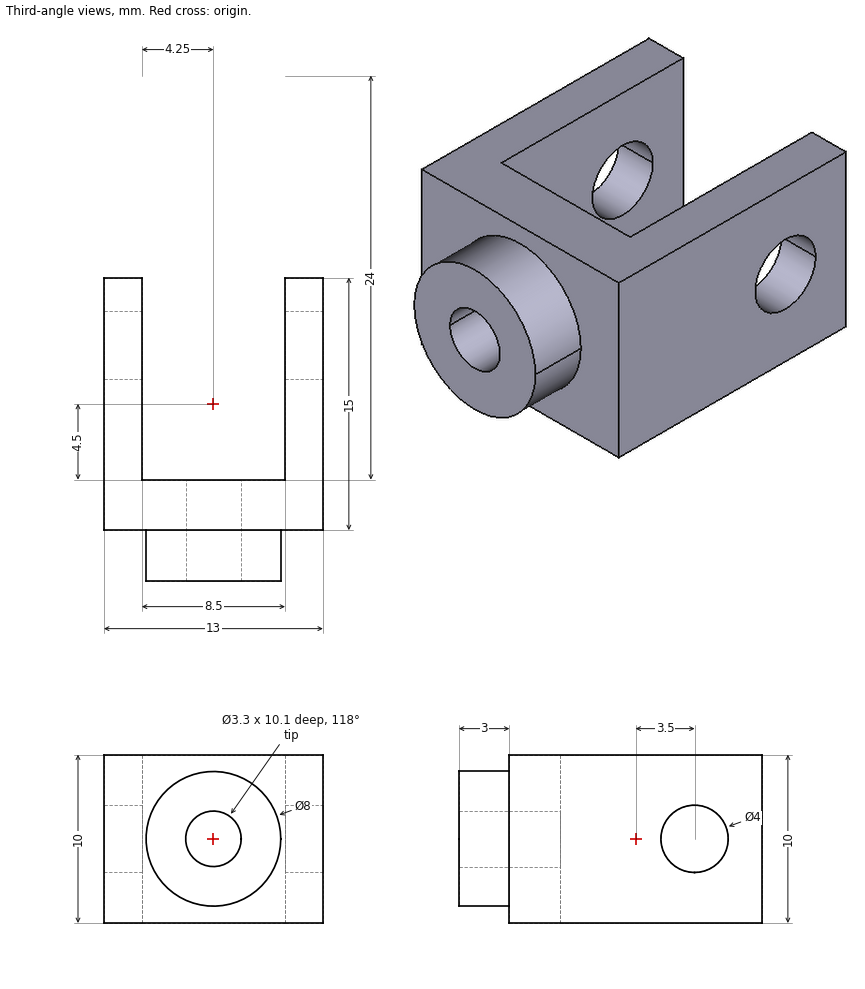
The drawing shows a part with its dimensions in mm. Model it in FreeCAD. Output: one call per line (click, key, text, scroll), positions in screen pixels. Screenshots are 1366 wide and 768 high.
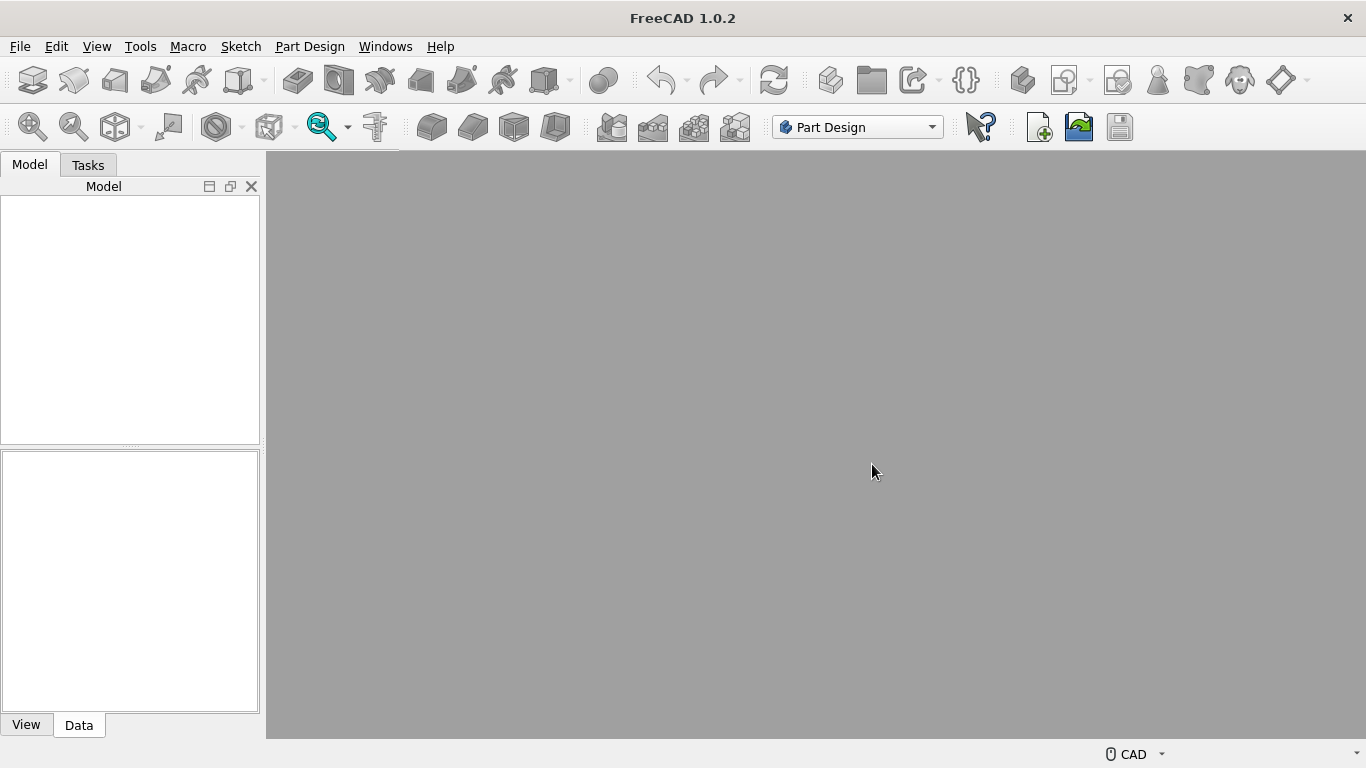
click(1038, 128)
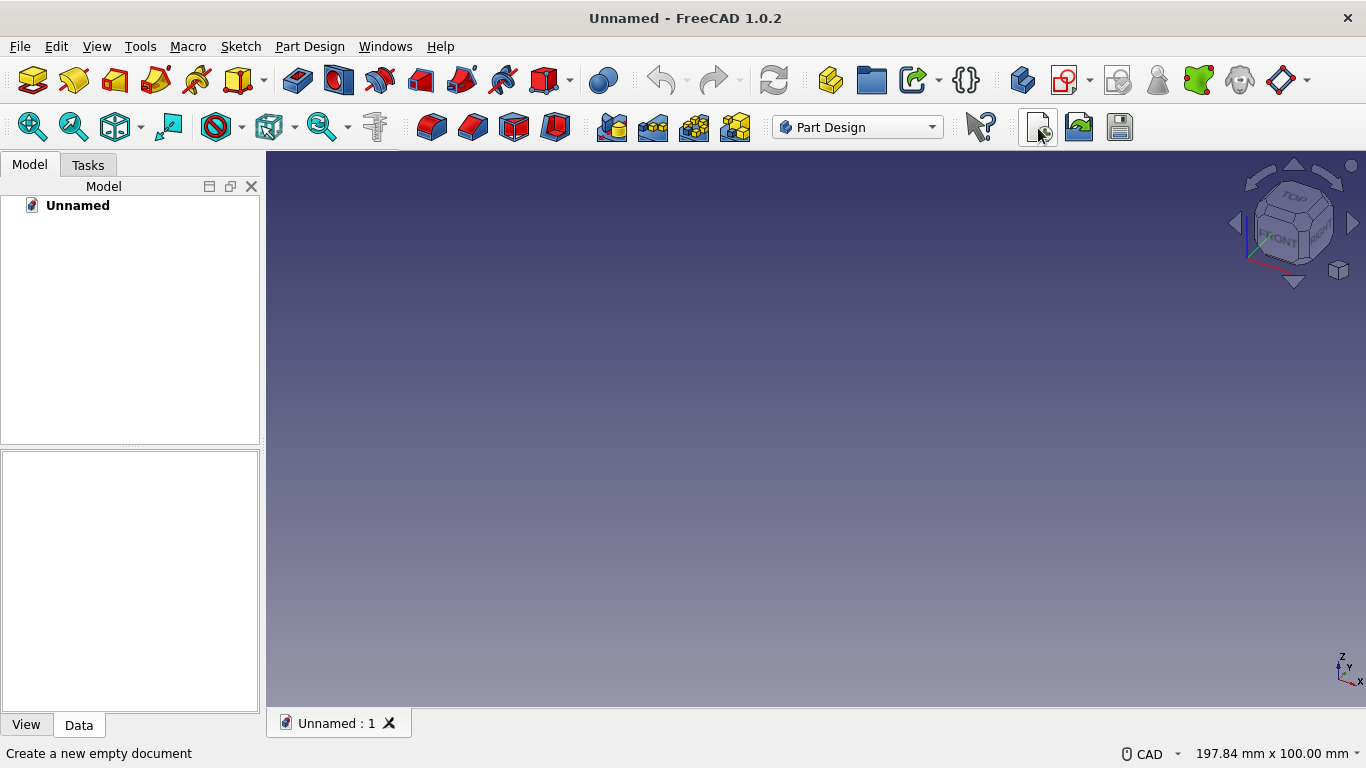
click(1064, 80)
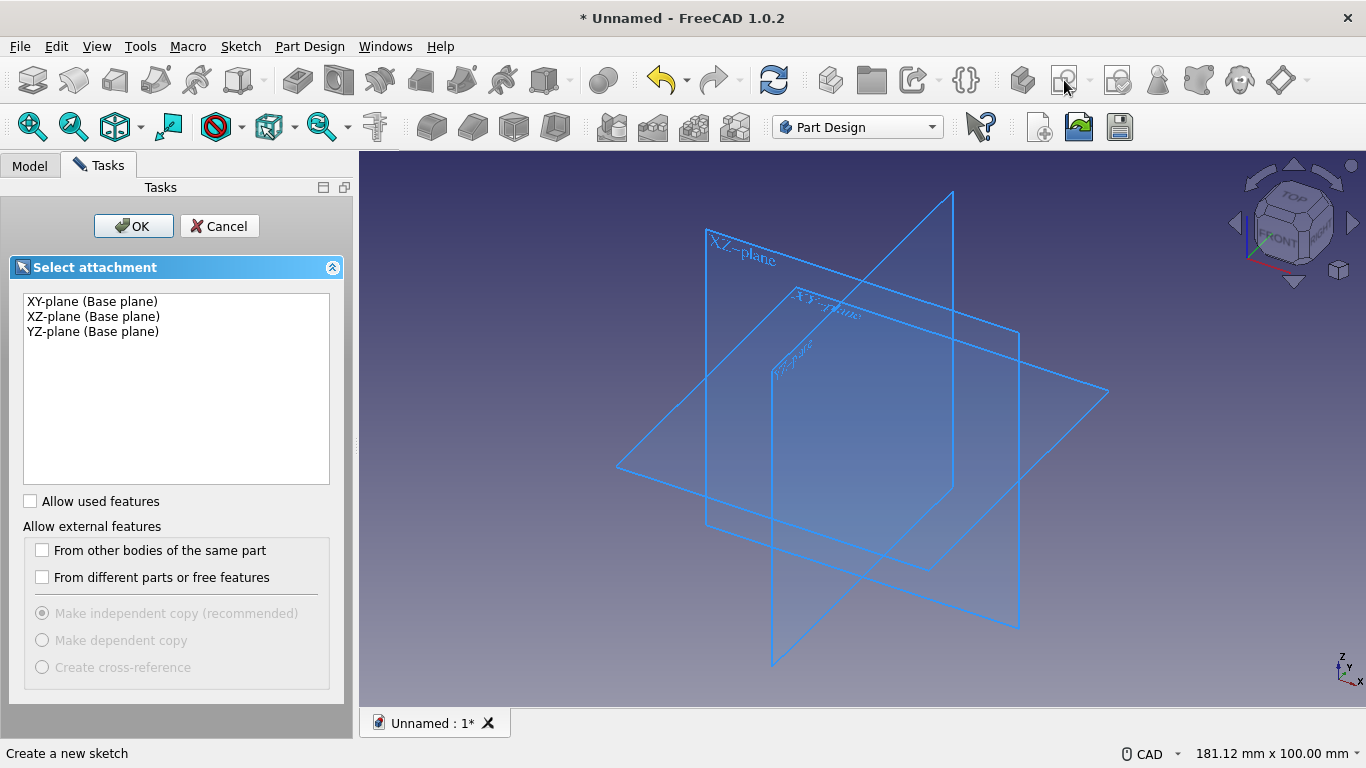
click(84, 302)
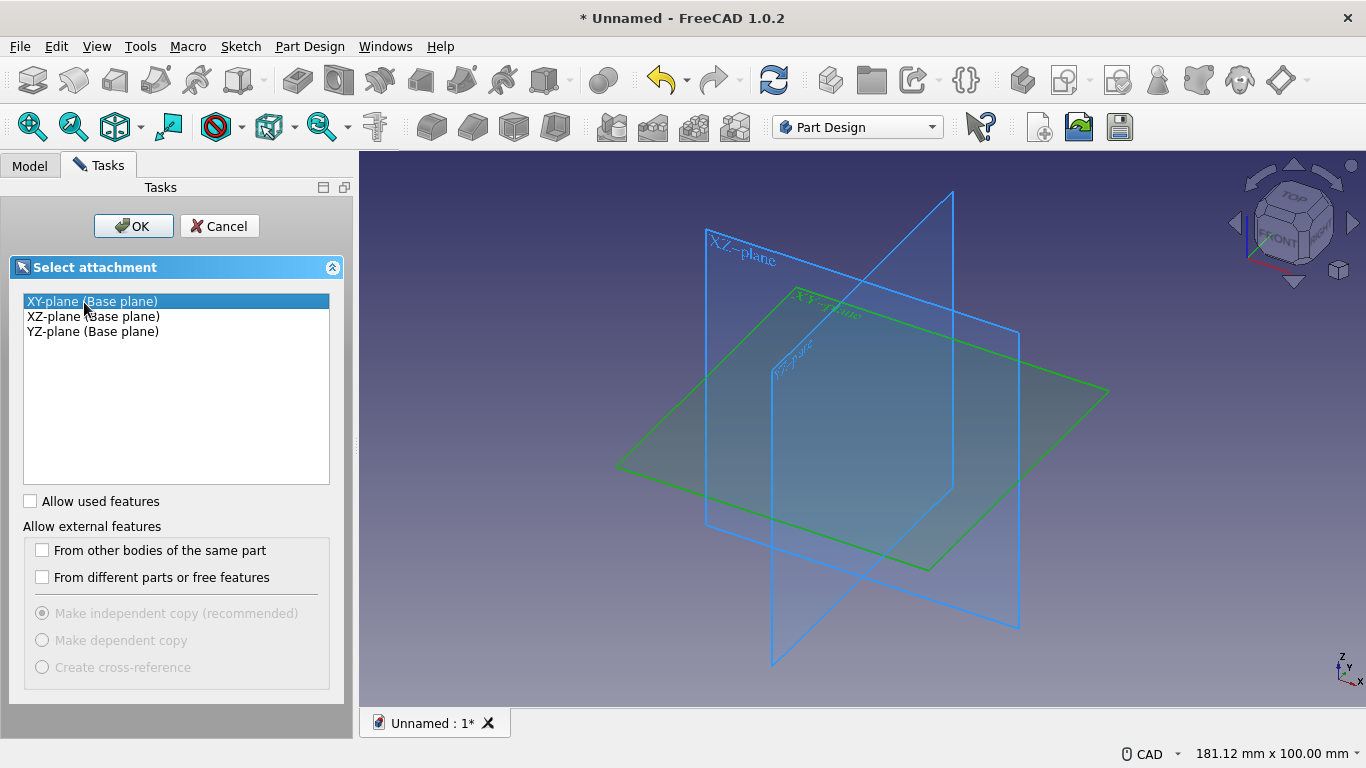
click(134, 226)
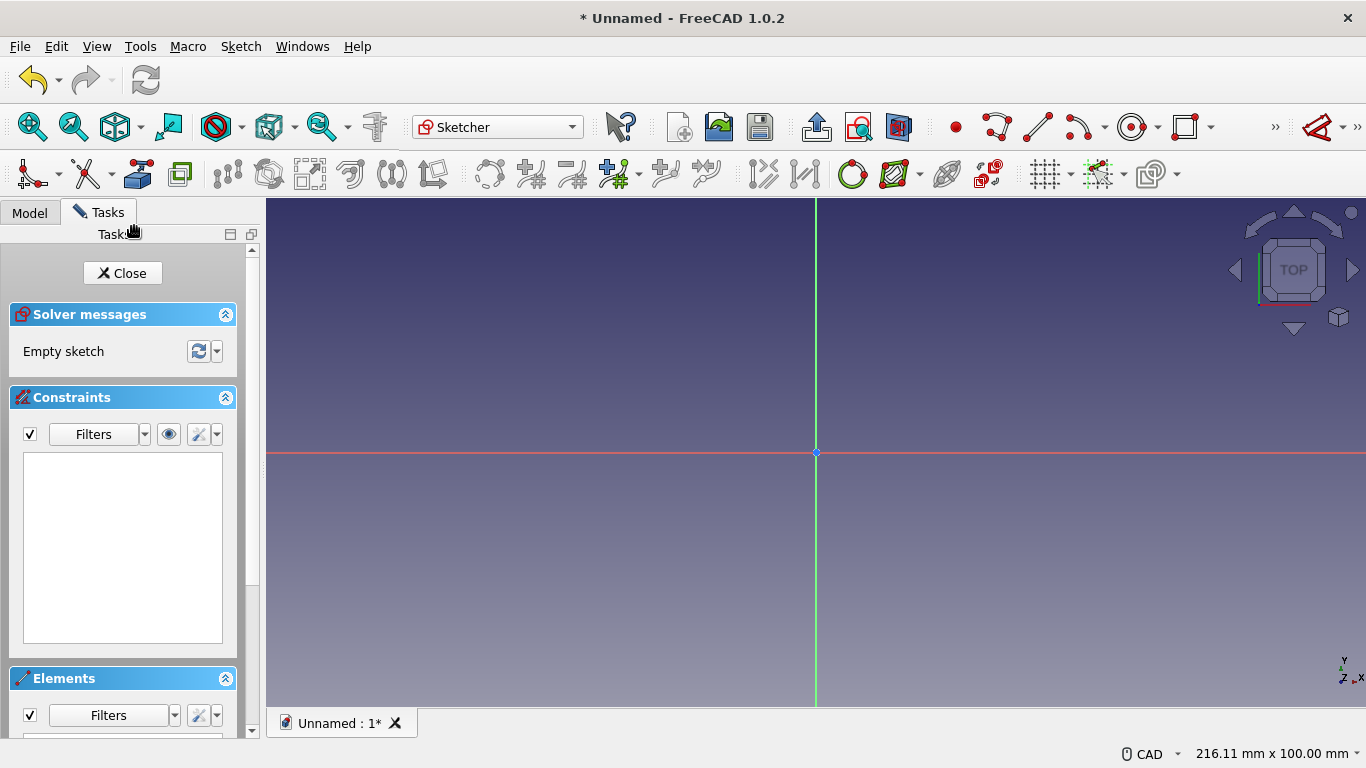
scroll(838, 452, up, 7)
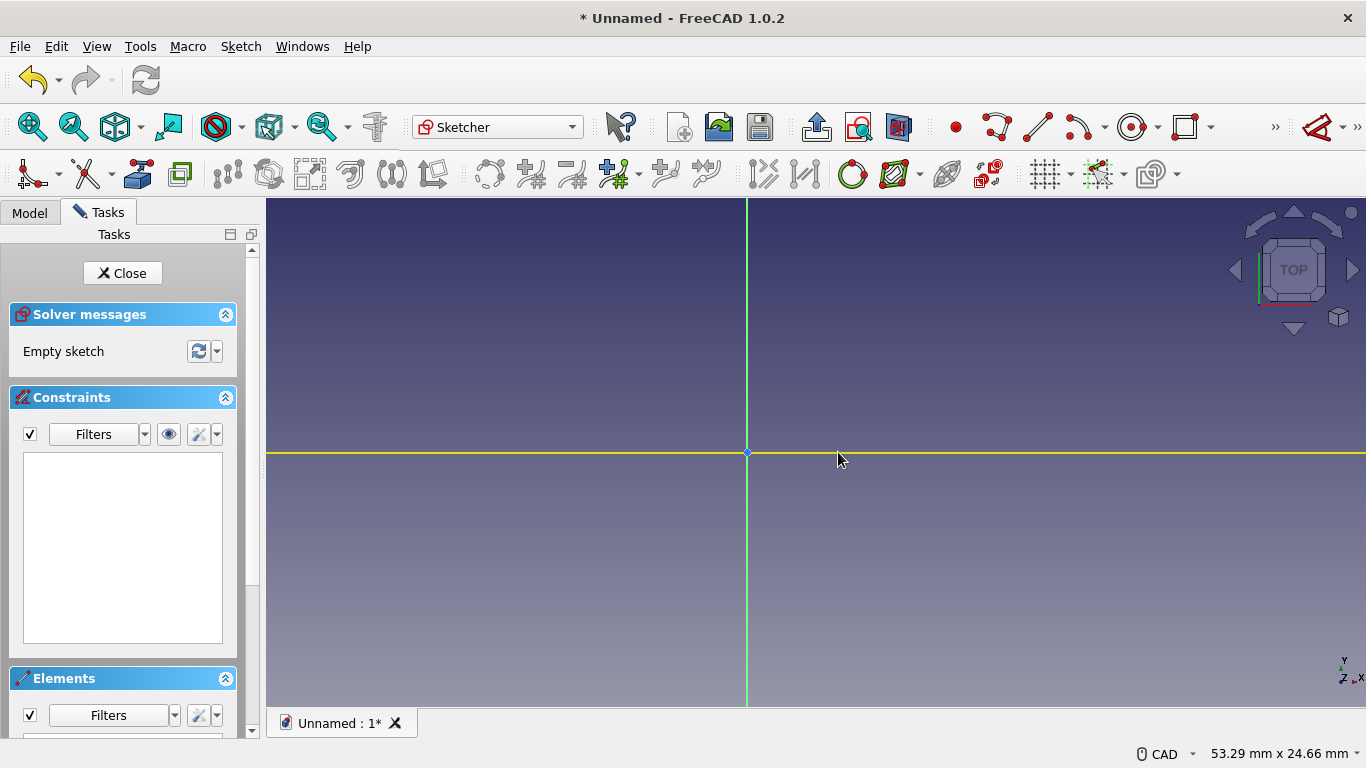
key(g)
key(v)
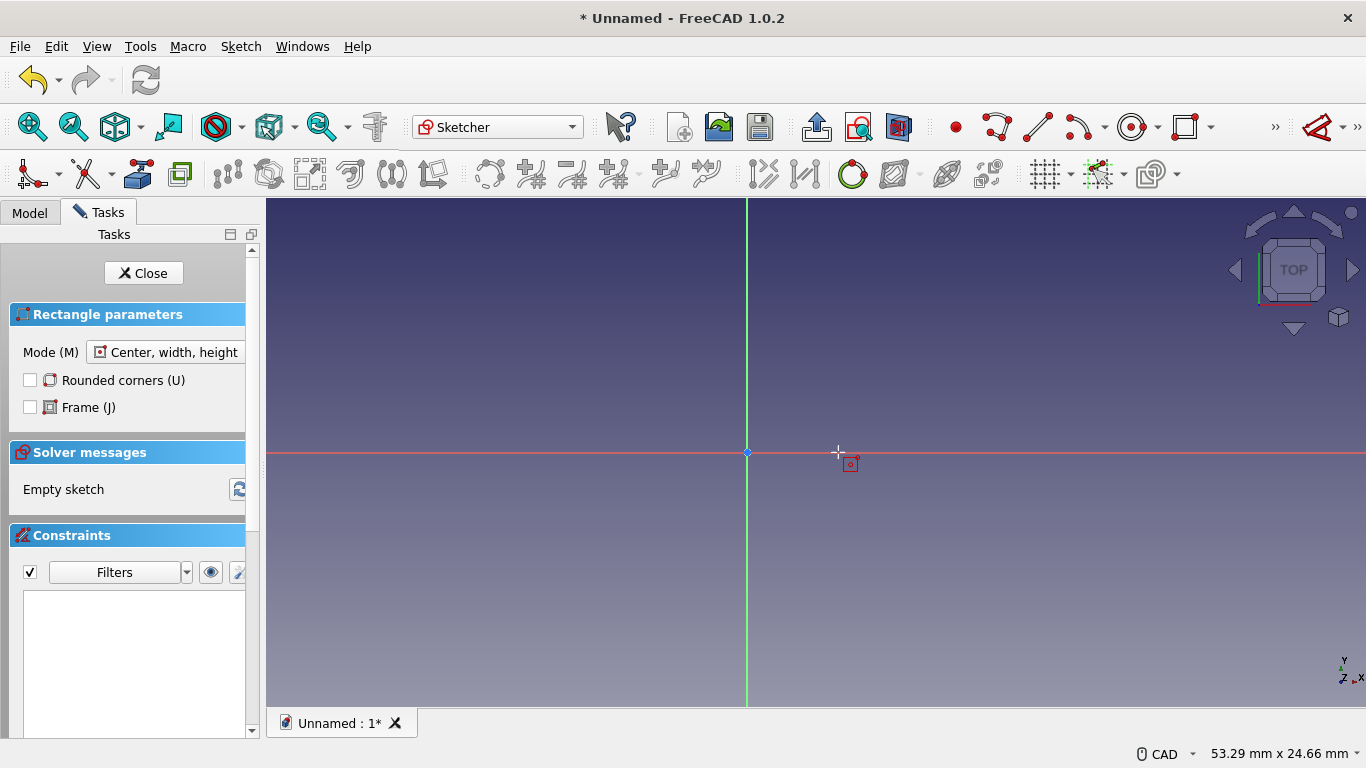
click(747, 452)
move(881, 298)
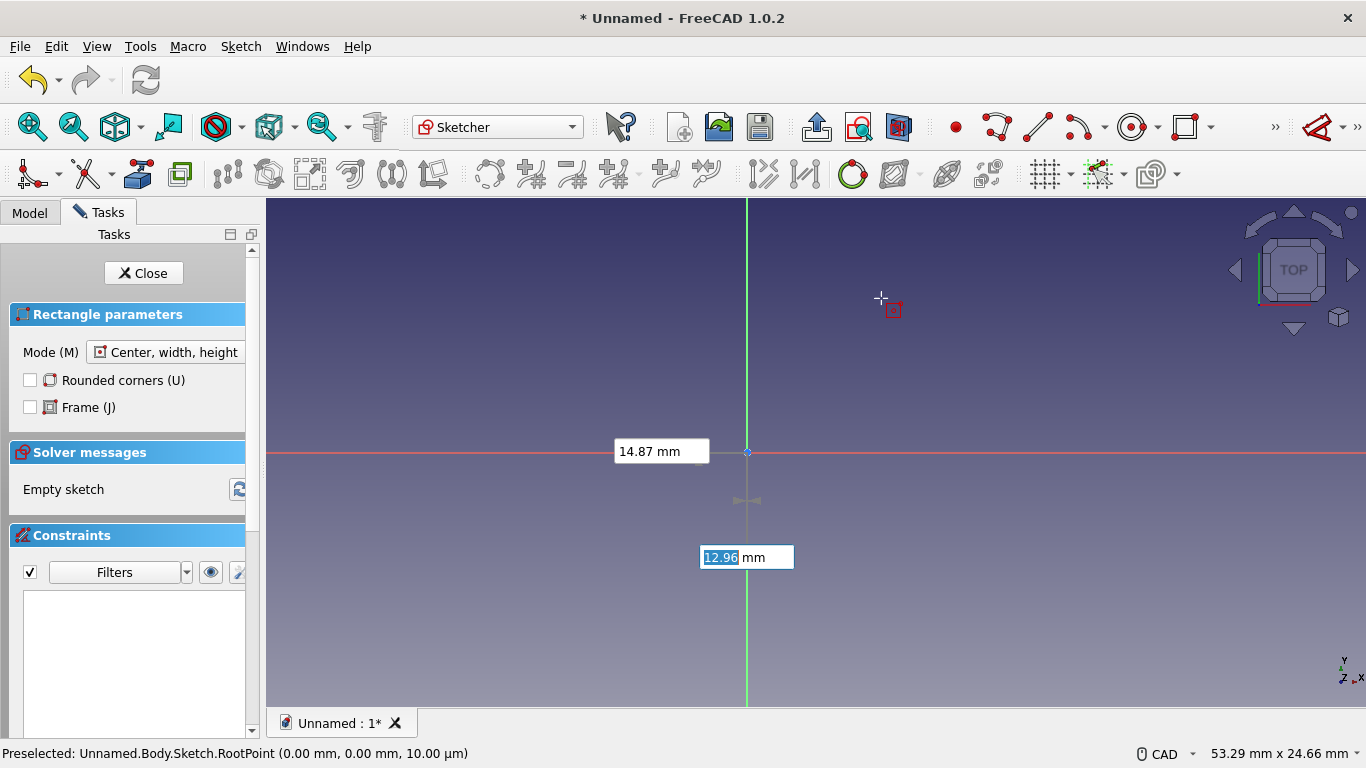
text(13)
key(Tab)
text(15)
key(Return)
key(Escape)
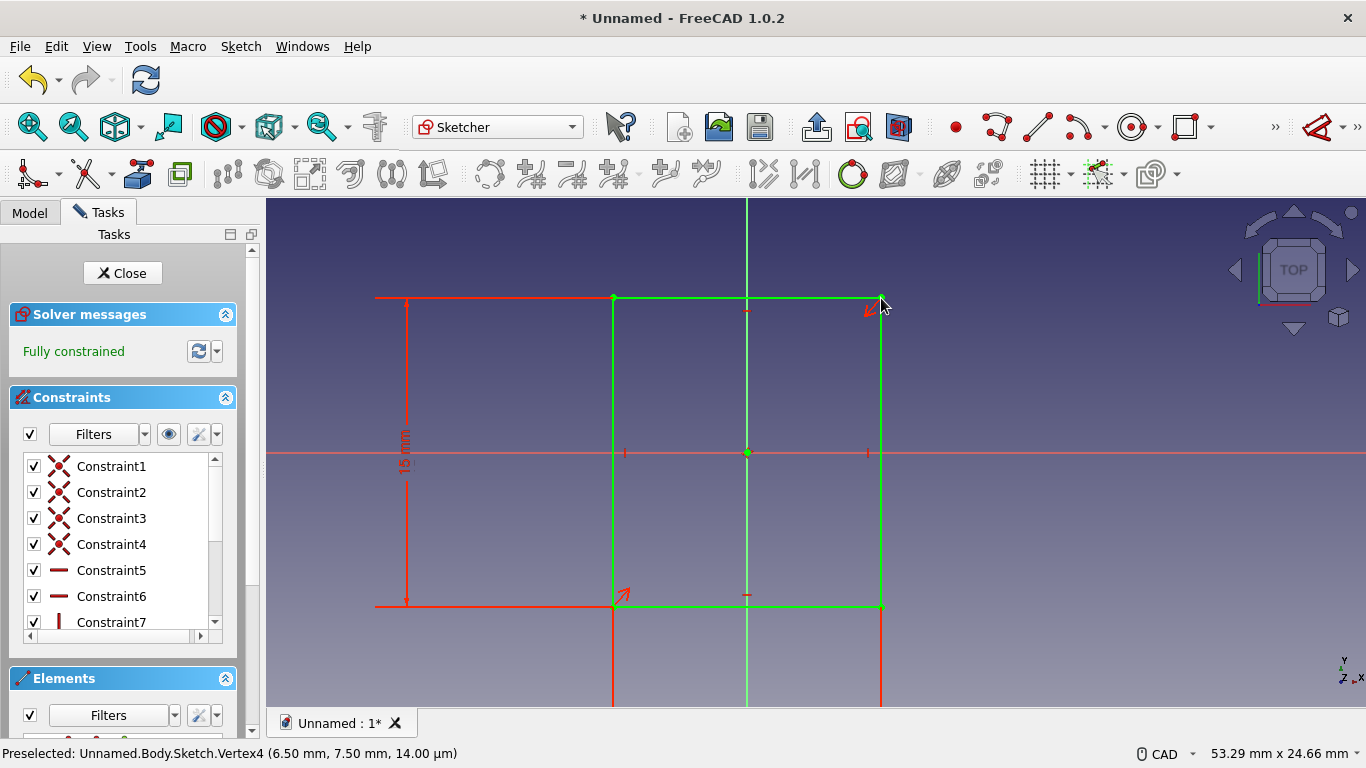
click(123, 273)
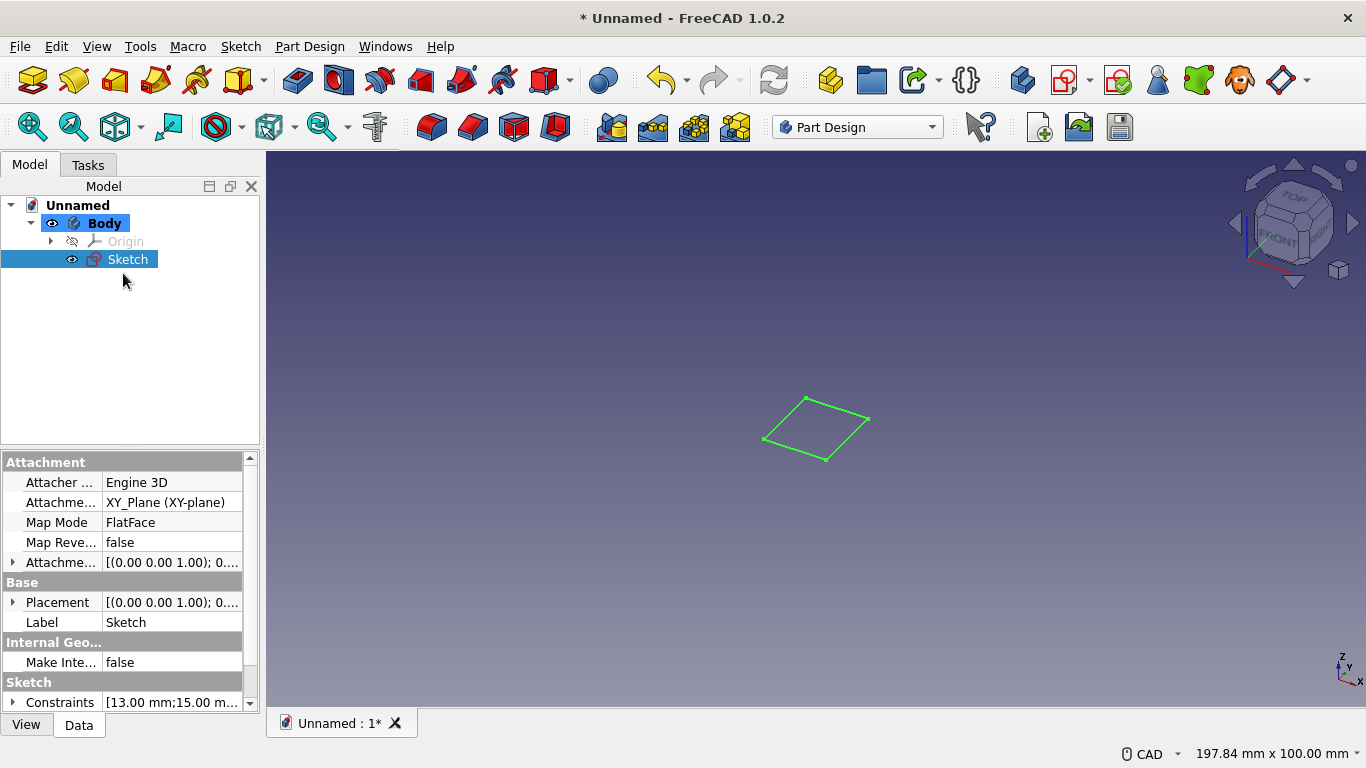
click(33, 80)